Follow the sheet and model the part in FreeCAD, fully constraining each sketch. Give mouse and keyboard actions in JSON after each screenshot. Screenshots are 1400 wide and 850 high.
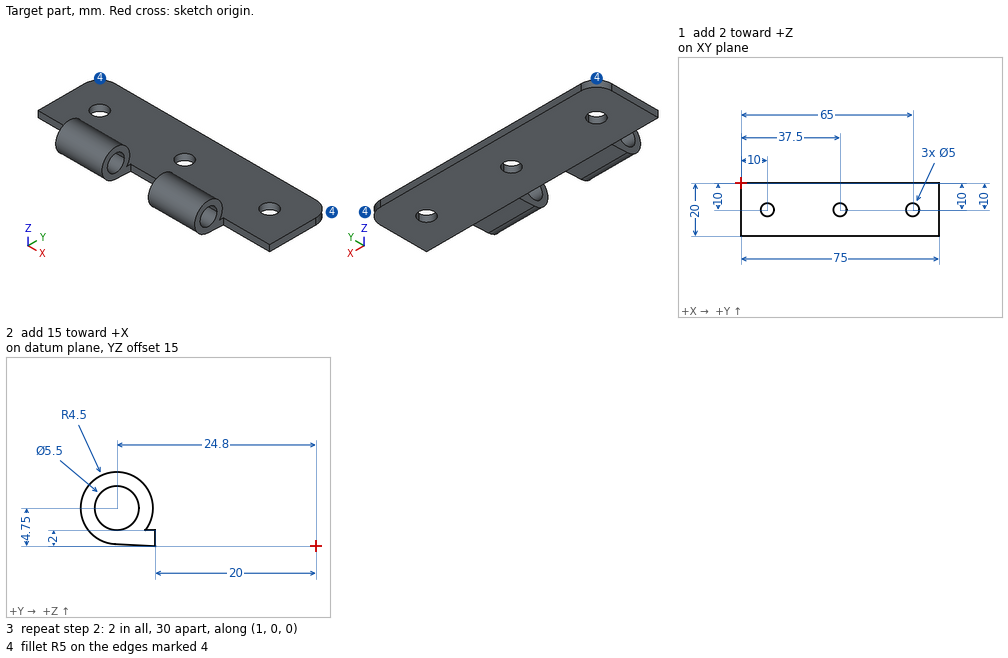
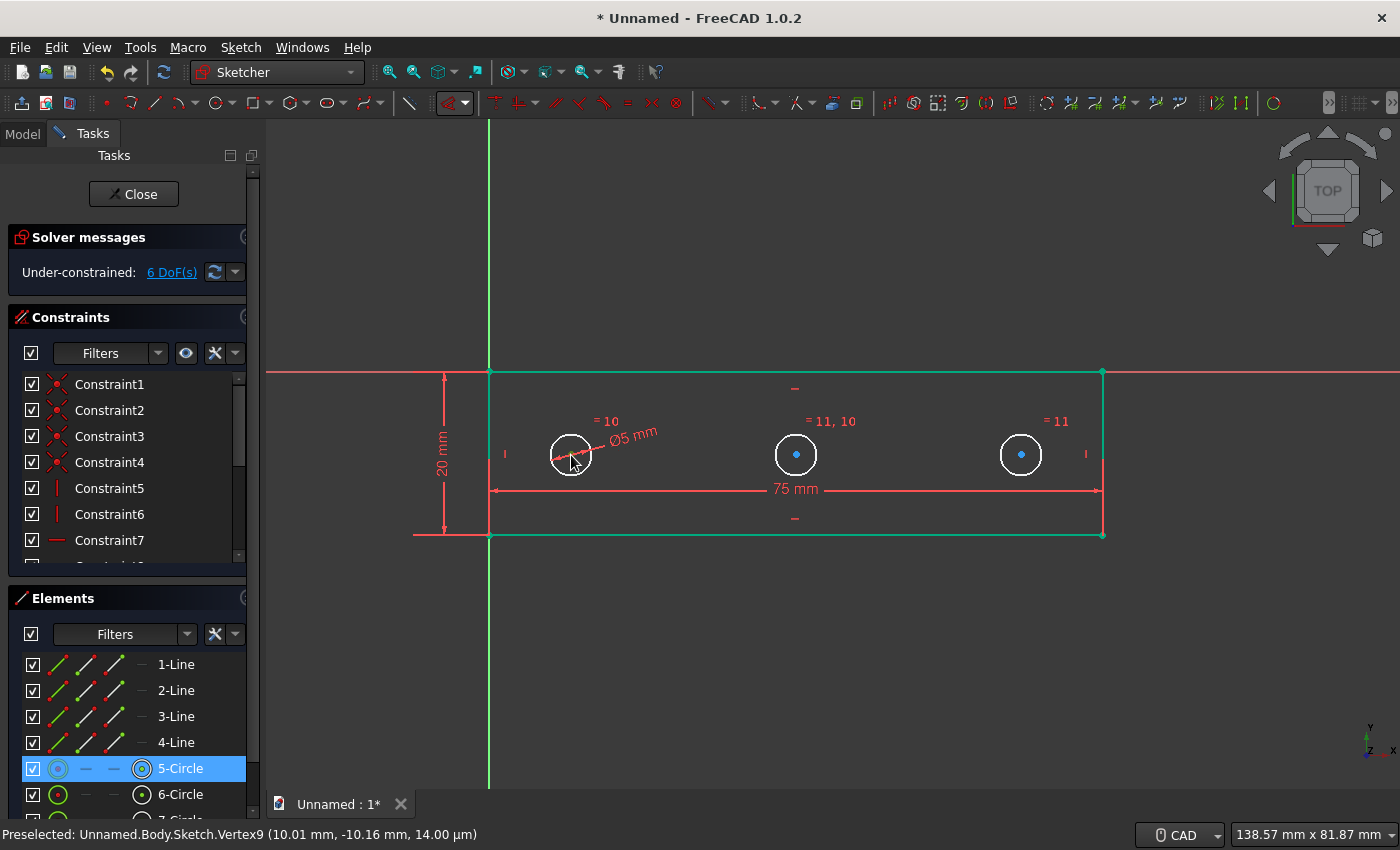
{"action": "key", "text": "l"}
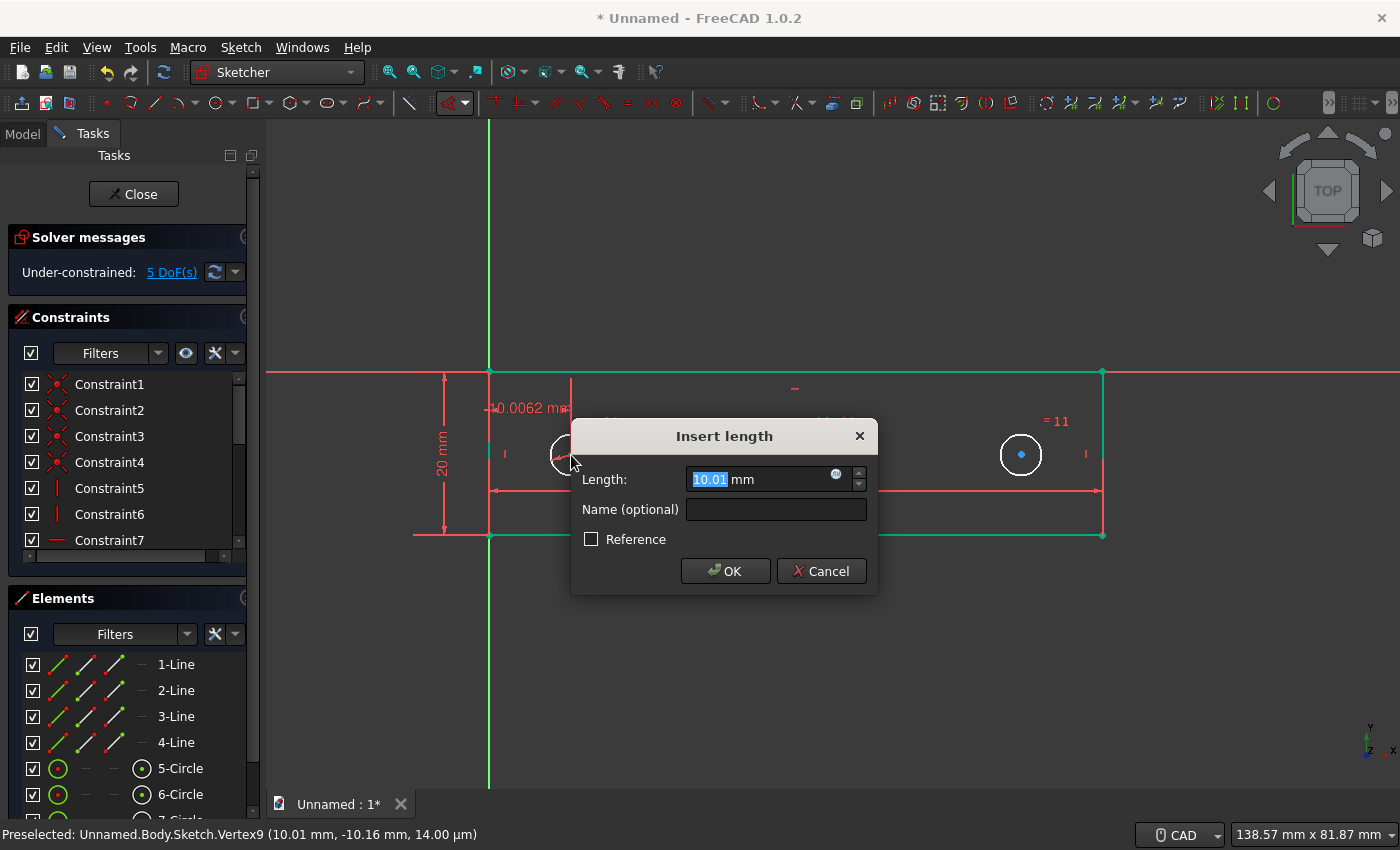
{"action": "type", "text": "10"}
{"action": "key", "text": "Return"}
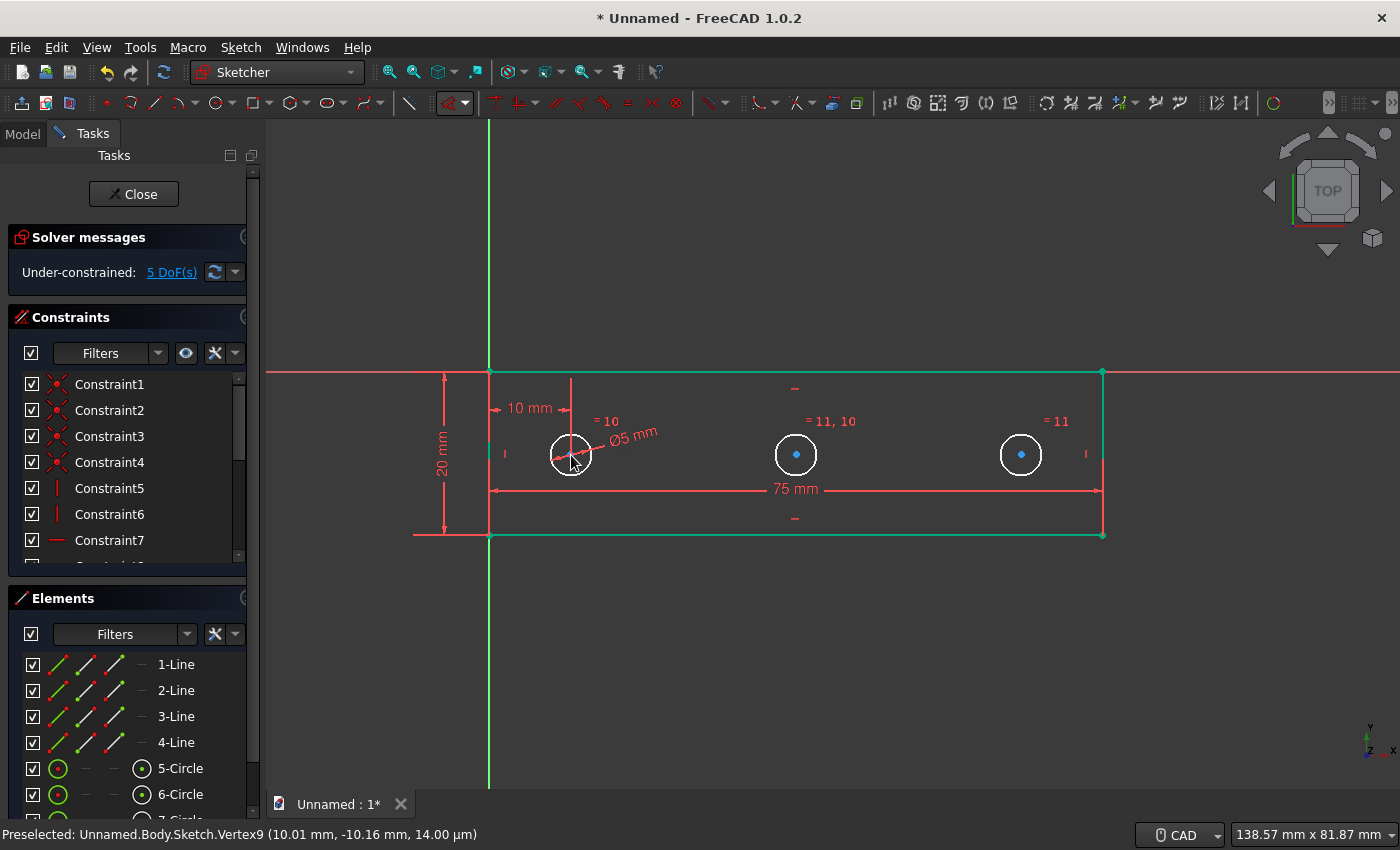
{"action": "left_click", "coordinate": [571, 455]}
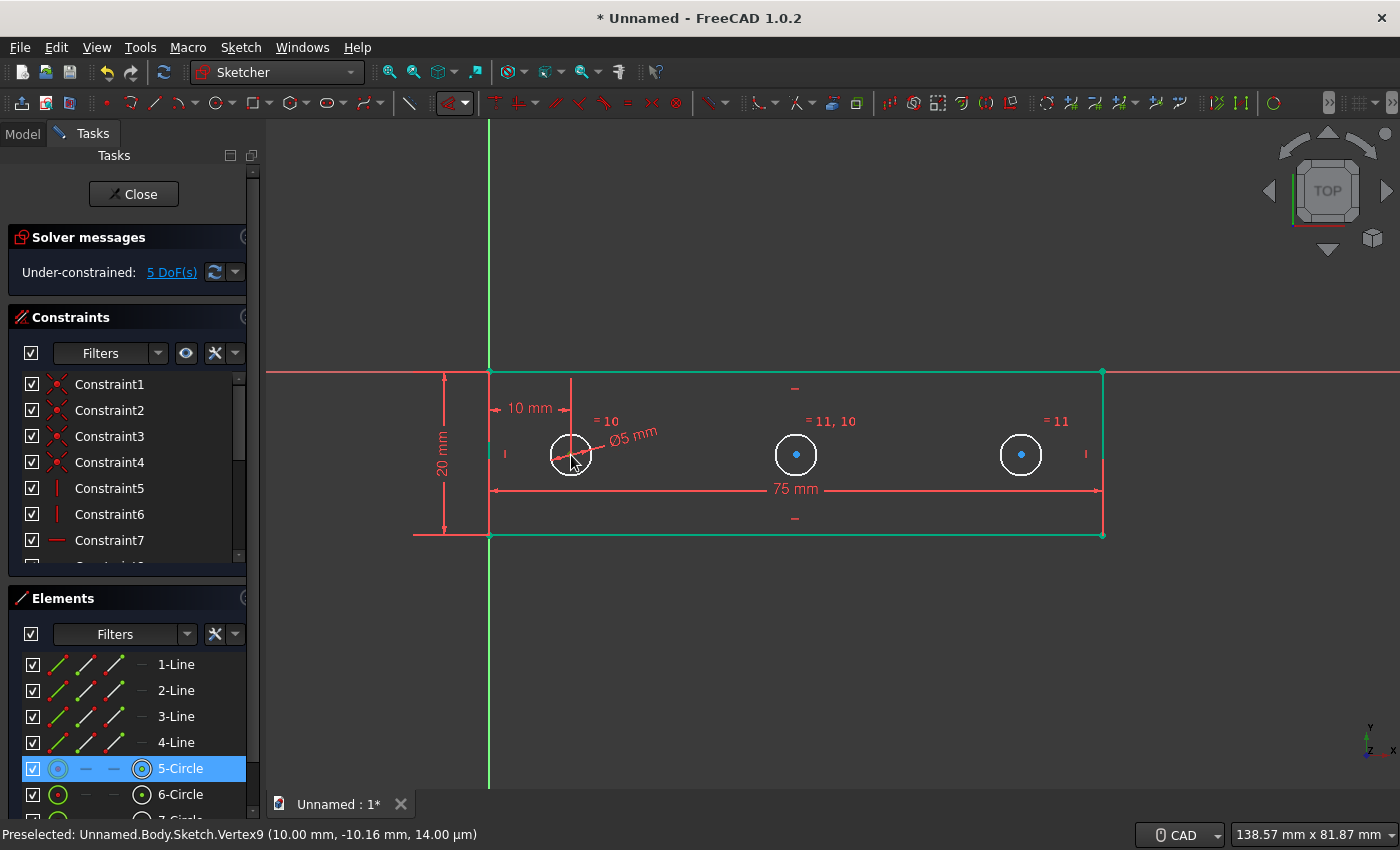
{"action": "left_click", "coordinate": [468, 104]}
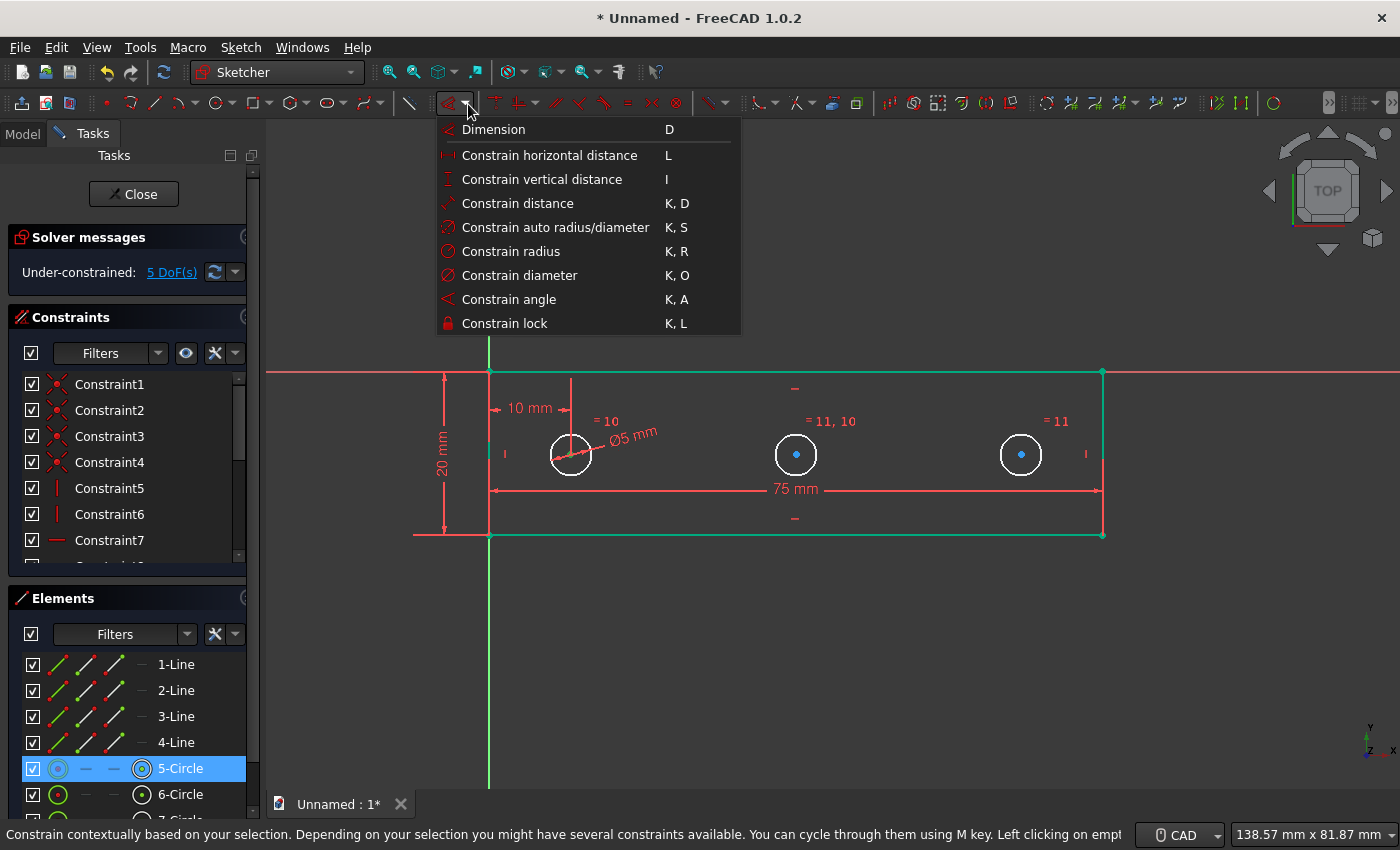
{"action": "left_click", "coordinate": [589, 179]}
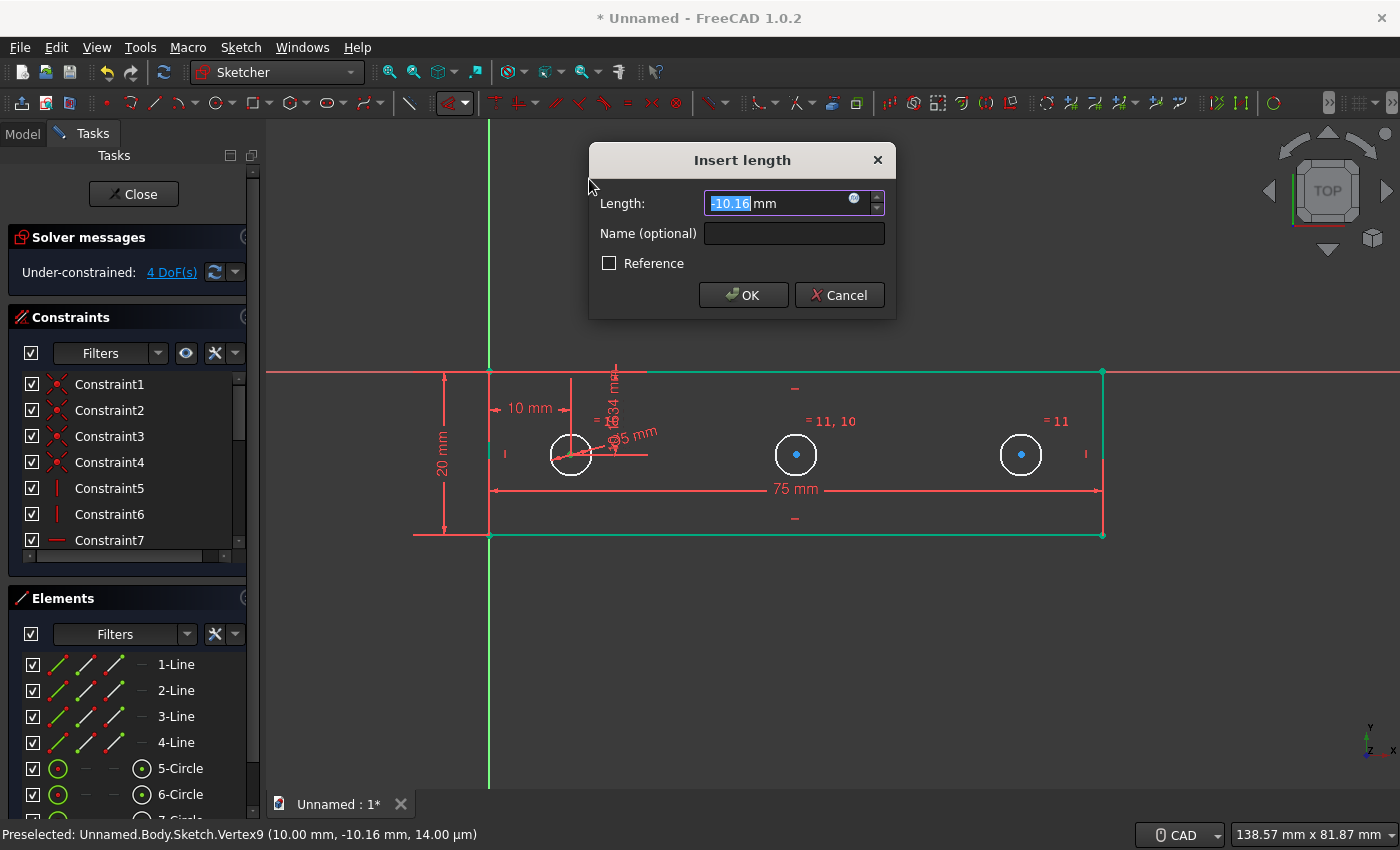
{"action": "type", "text": "-10"}
{"action": "key", "text": "Return"}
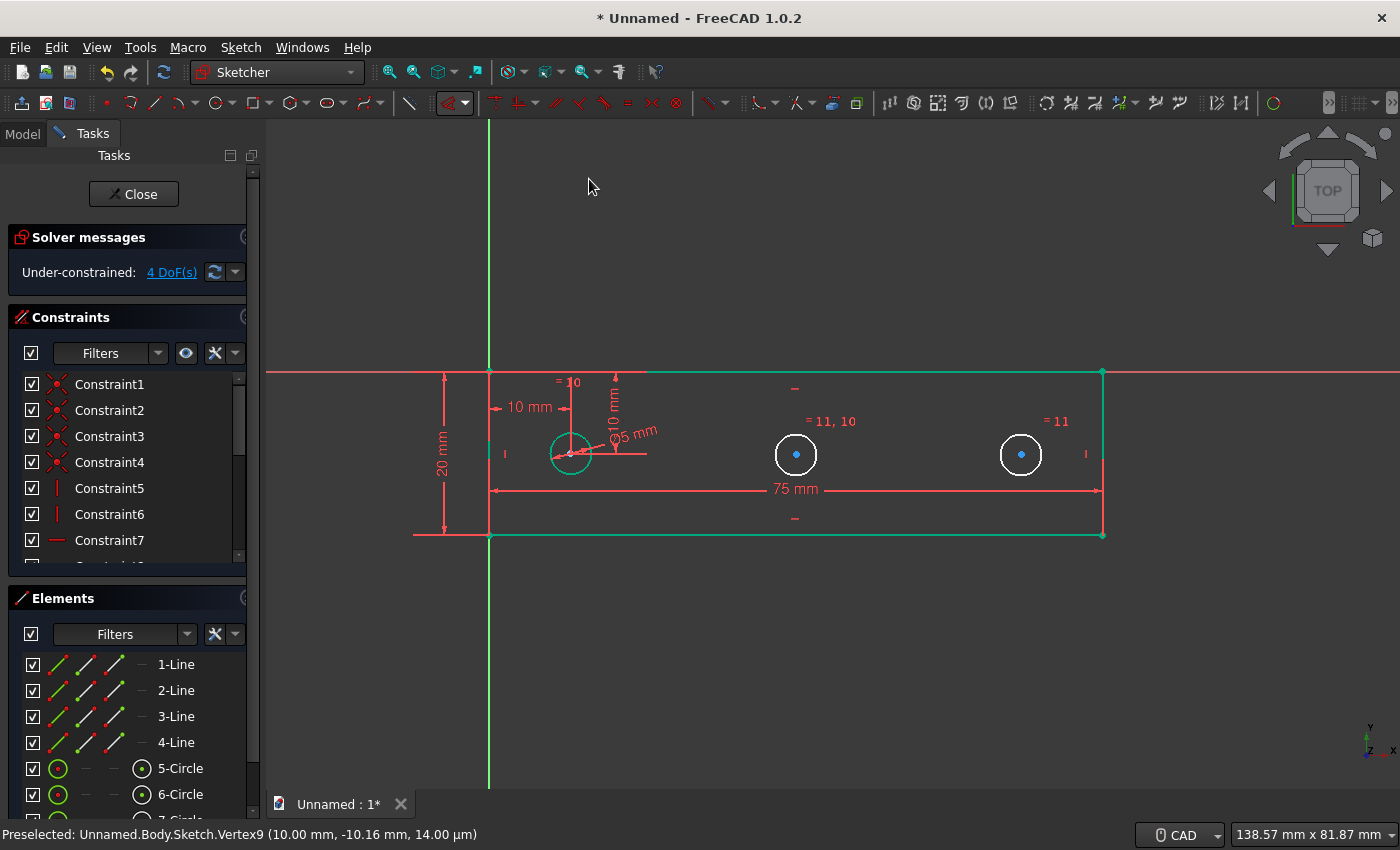
{"action": "left_click", "coordinate": [796, 455]}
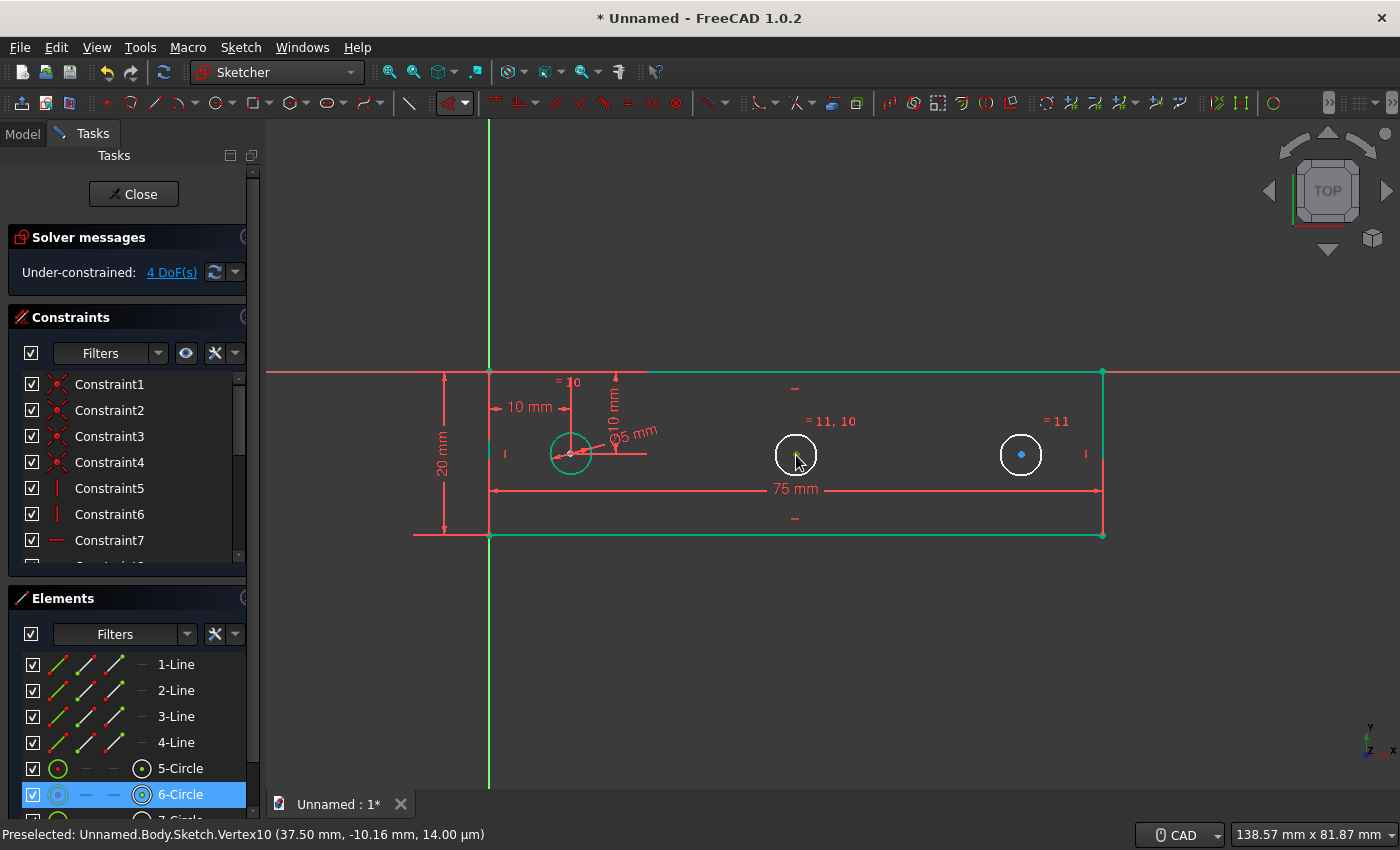
{"action": "left_click", "coordinate": [468, 104]}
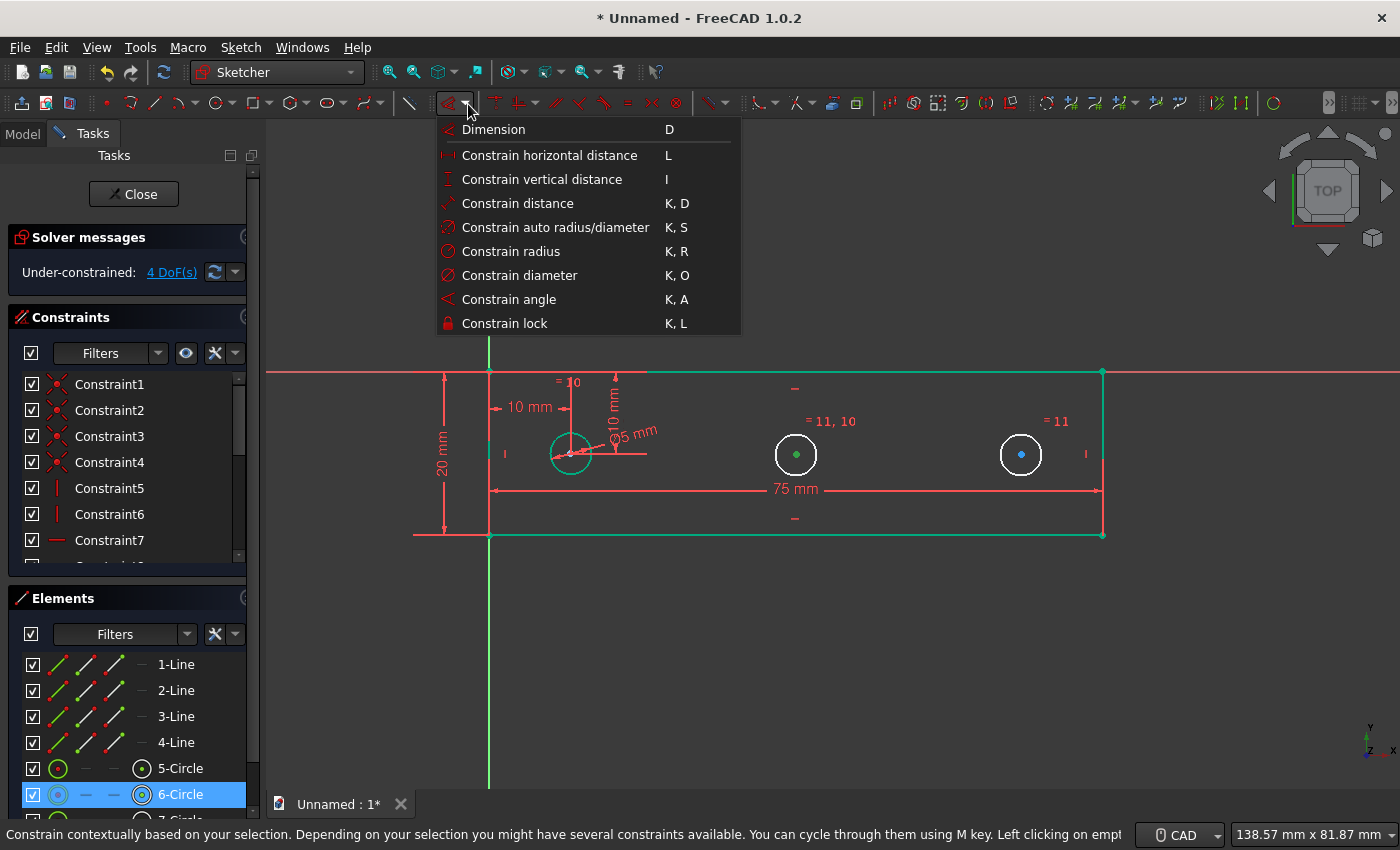
{"action": "left_click", "coordinate": [589, 179]}